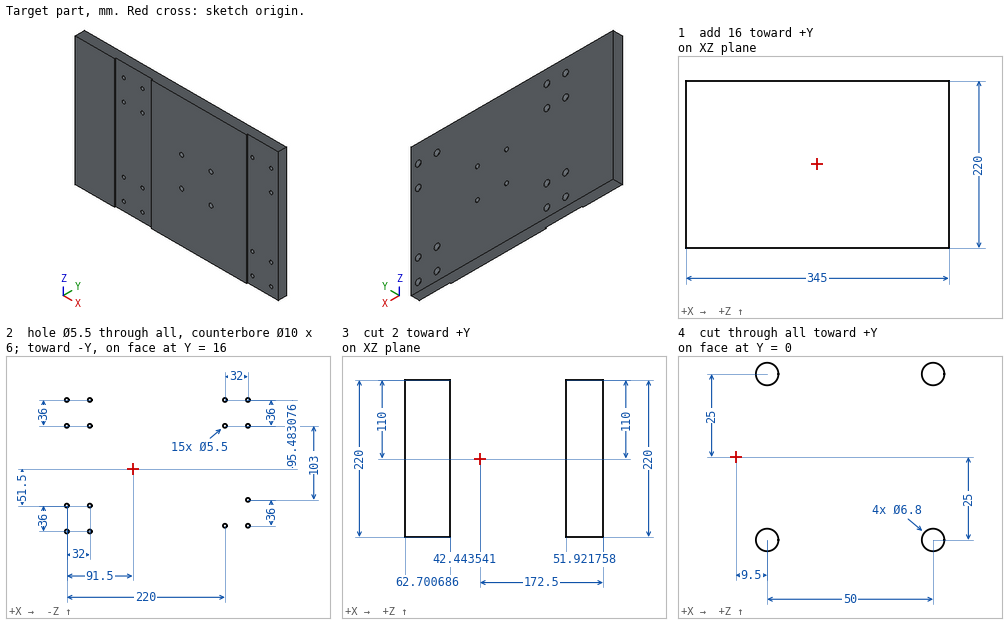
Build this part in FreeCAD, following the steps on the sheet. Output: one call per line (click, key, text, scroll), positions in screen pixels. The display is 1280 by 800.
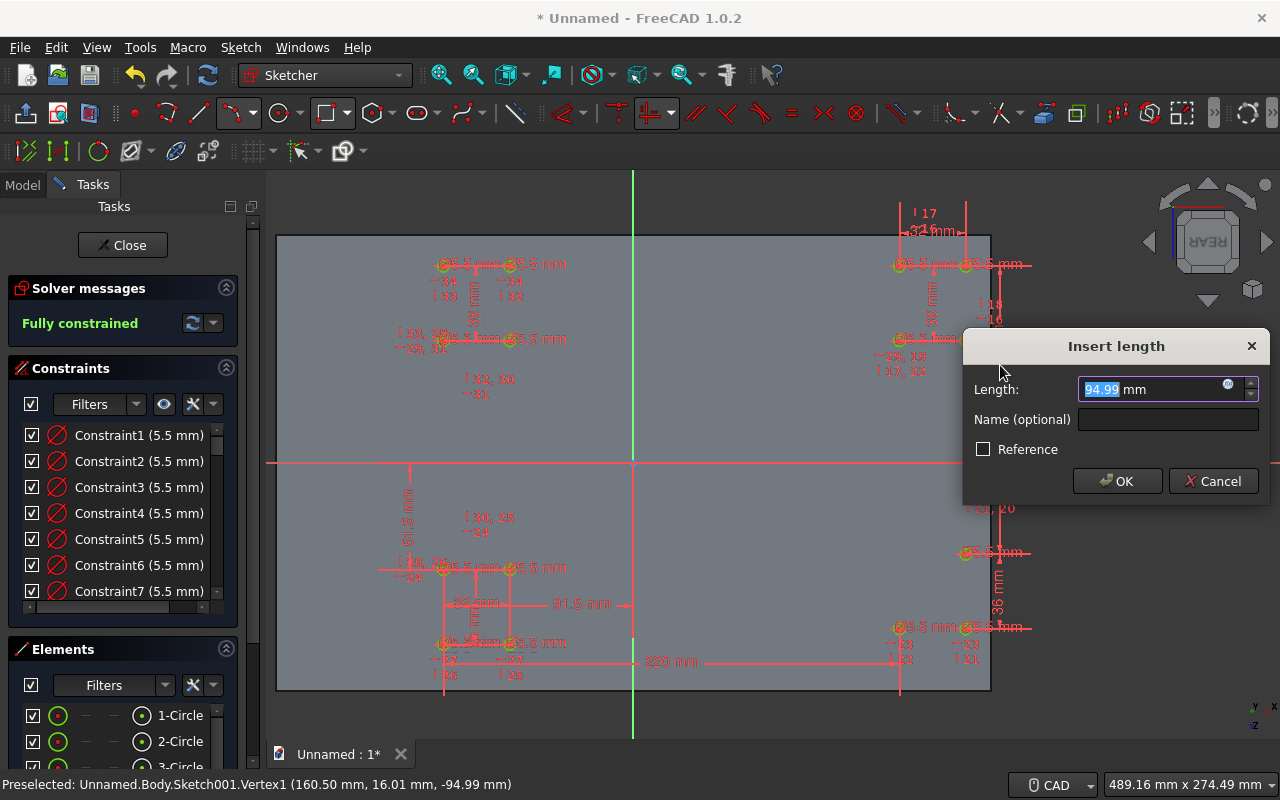
text(95.483076)
key(Return)
key(Escape)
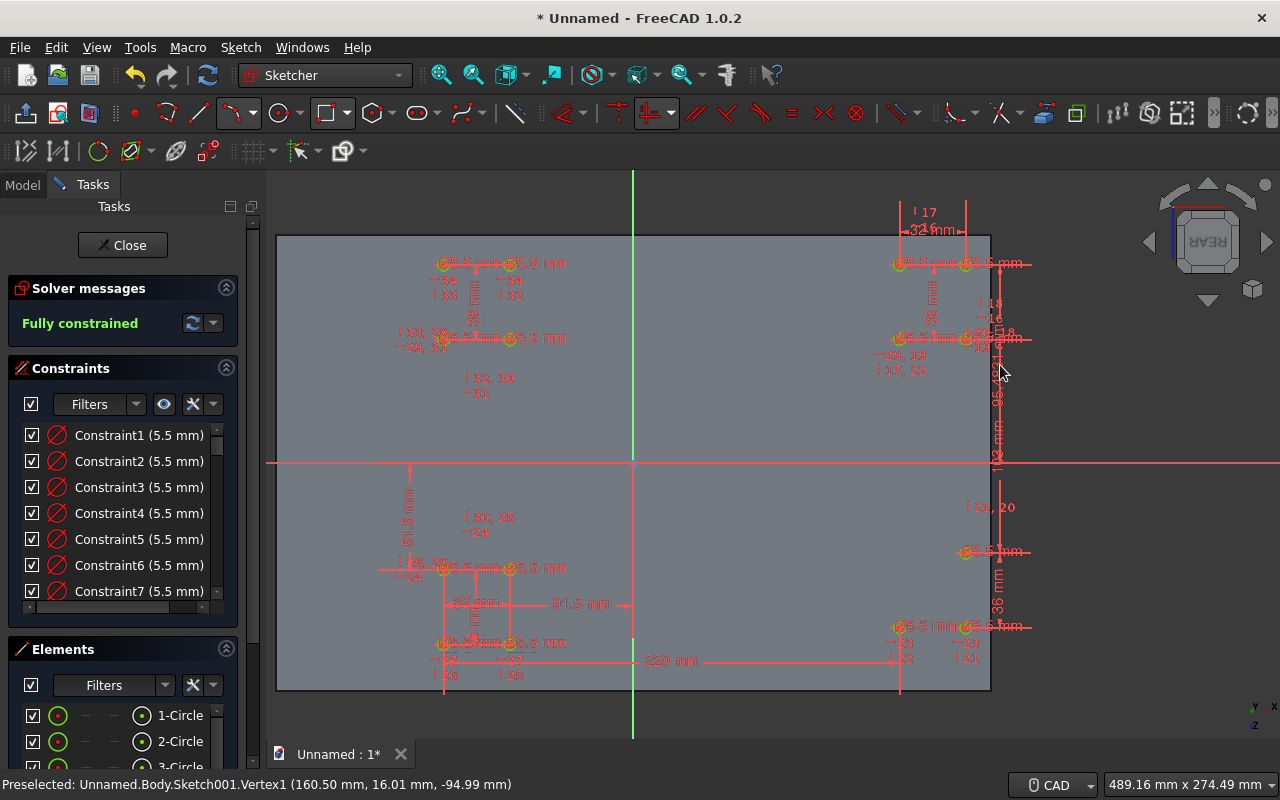
click(123, 245)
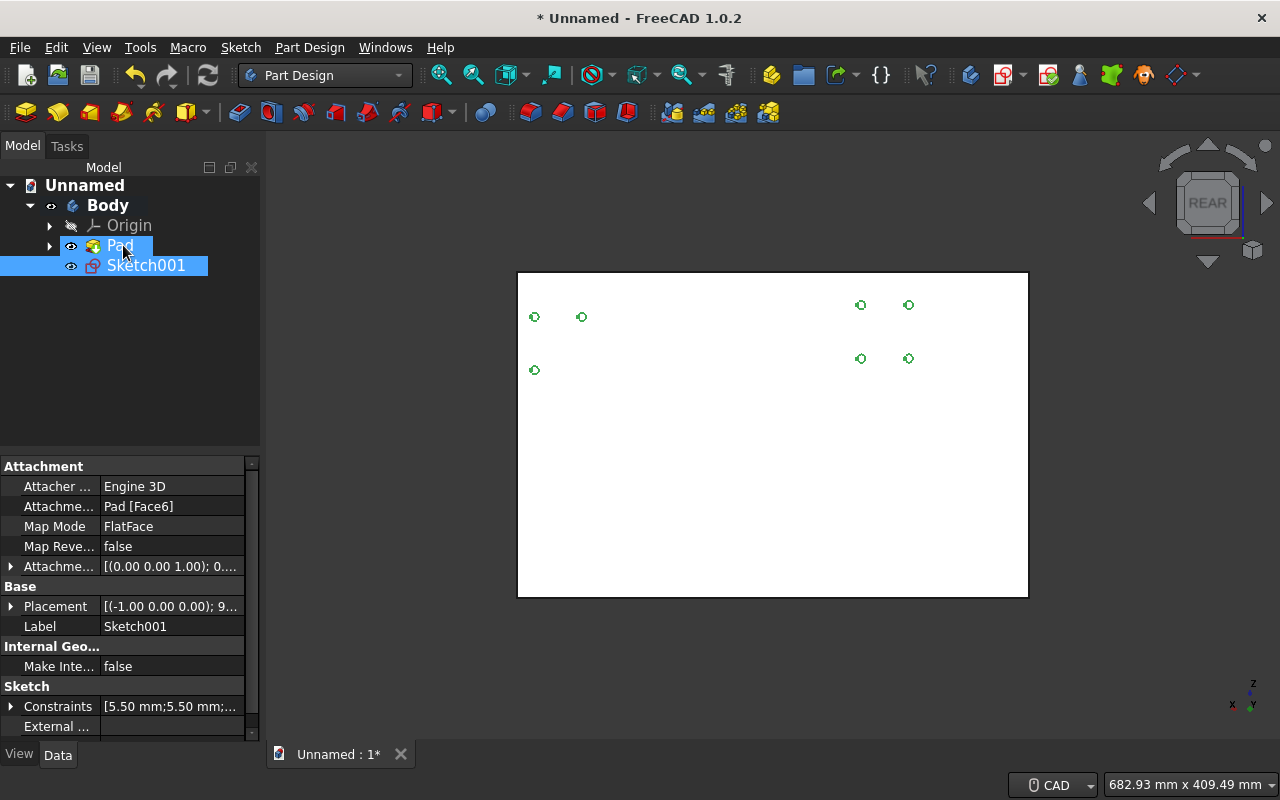
click(272, 112)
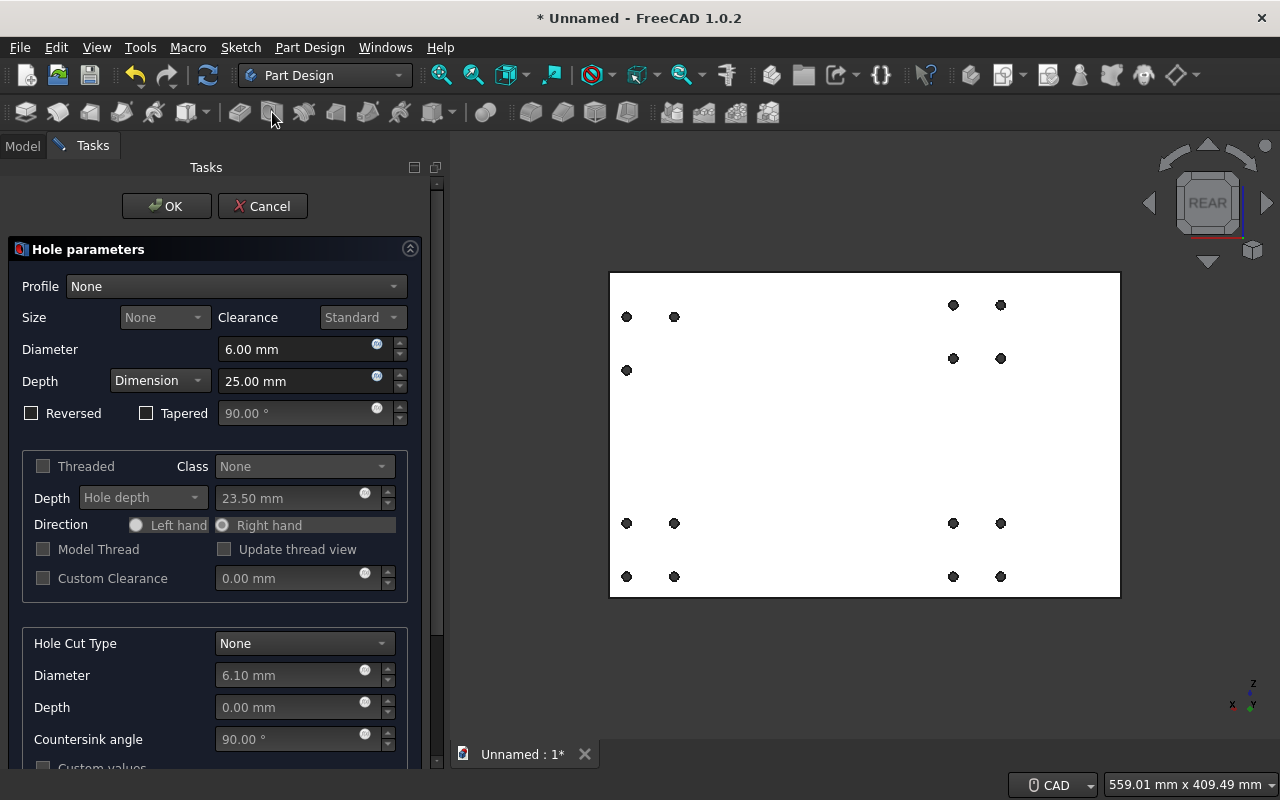
triple_click(305, 349)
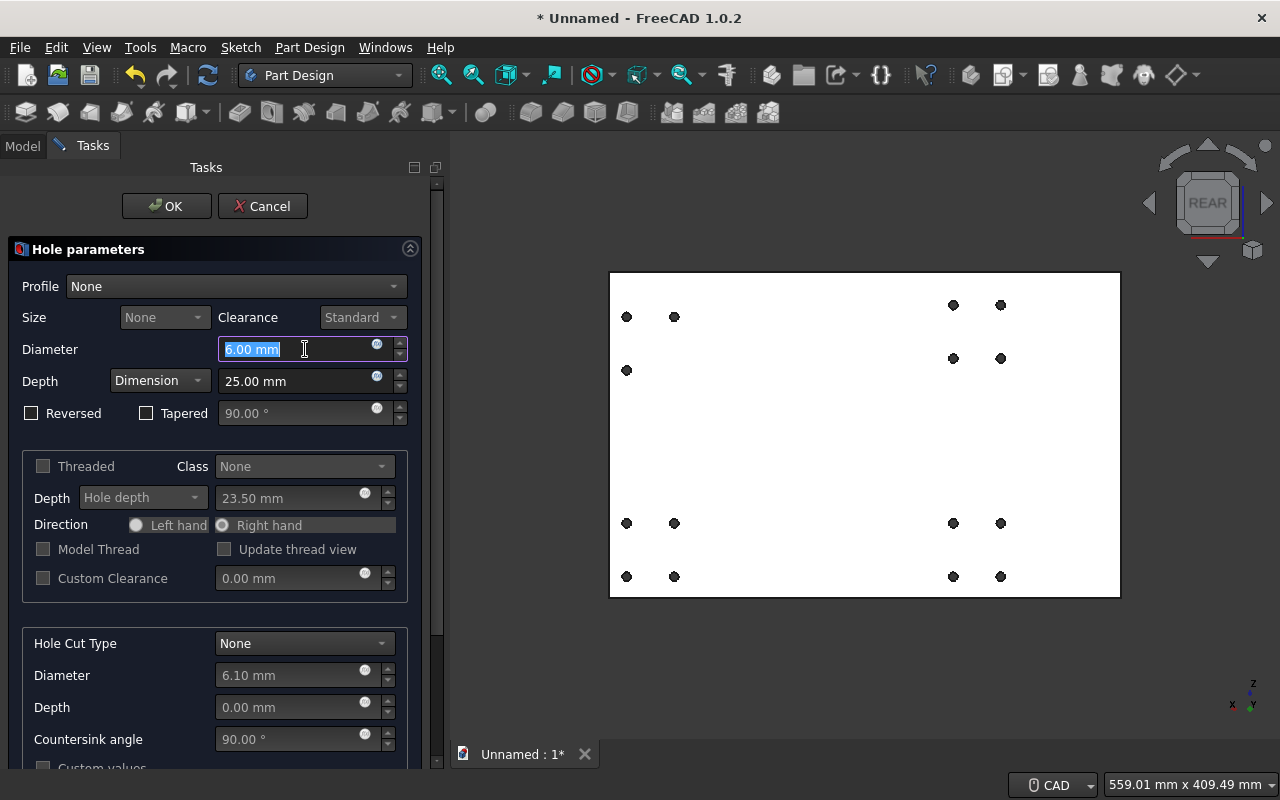
text(5.5)
key(Tab)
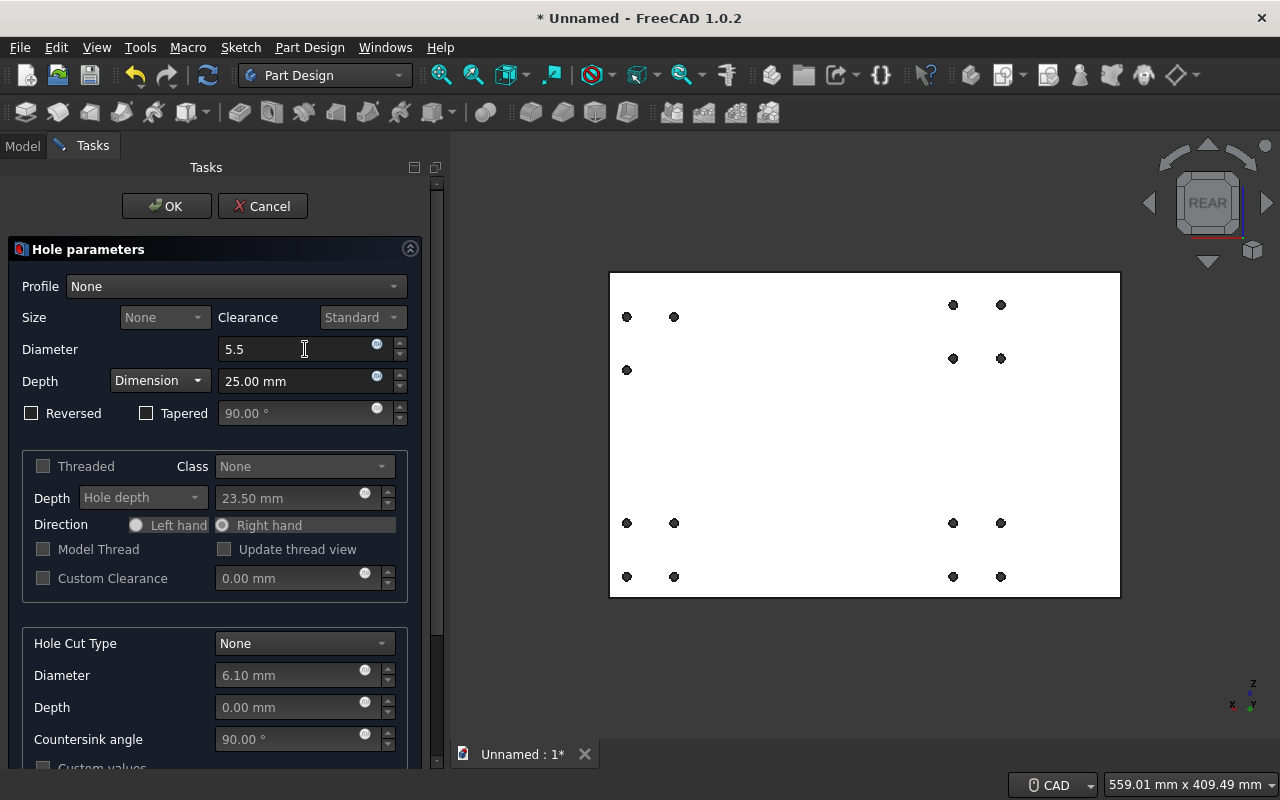
click(161, 380)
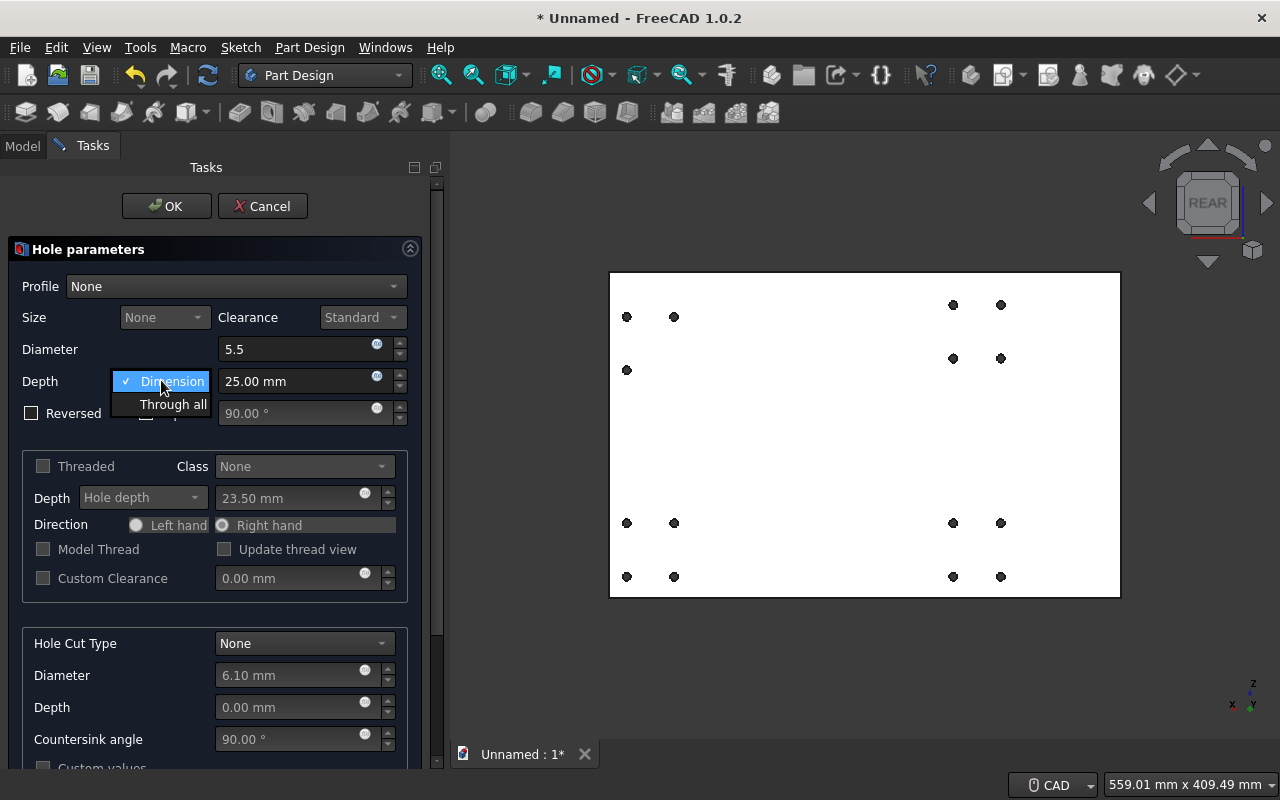
click(160, 404)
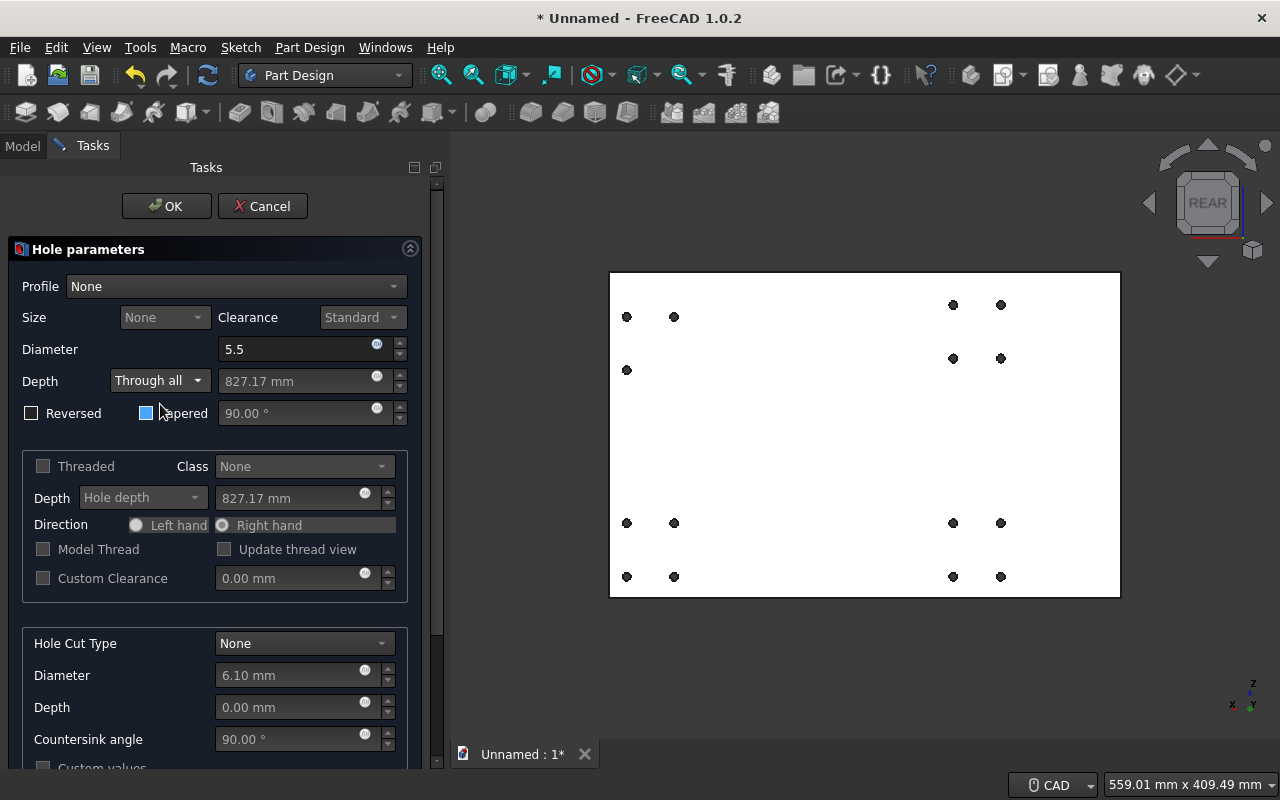
click(306, 644)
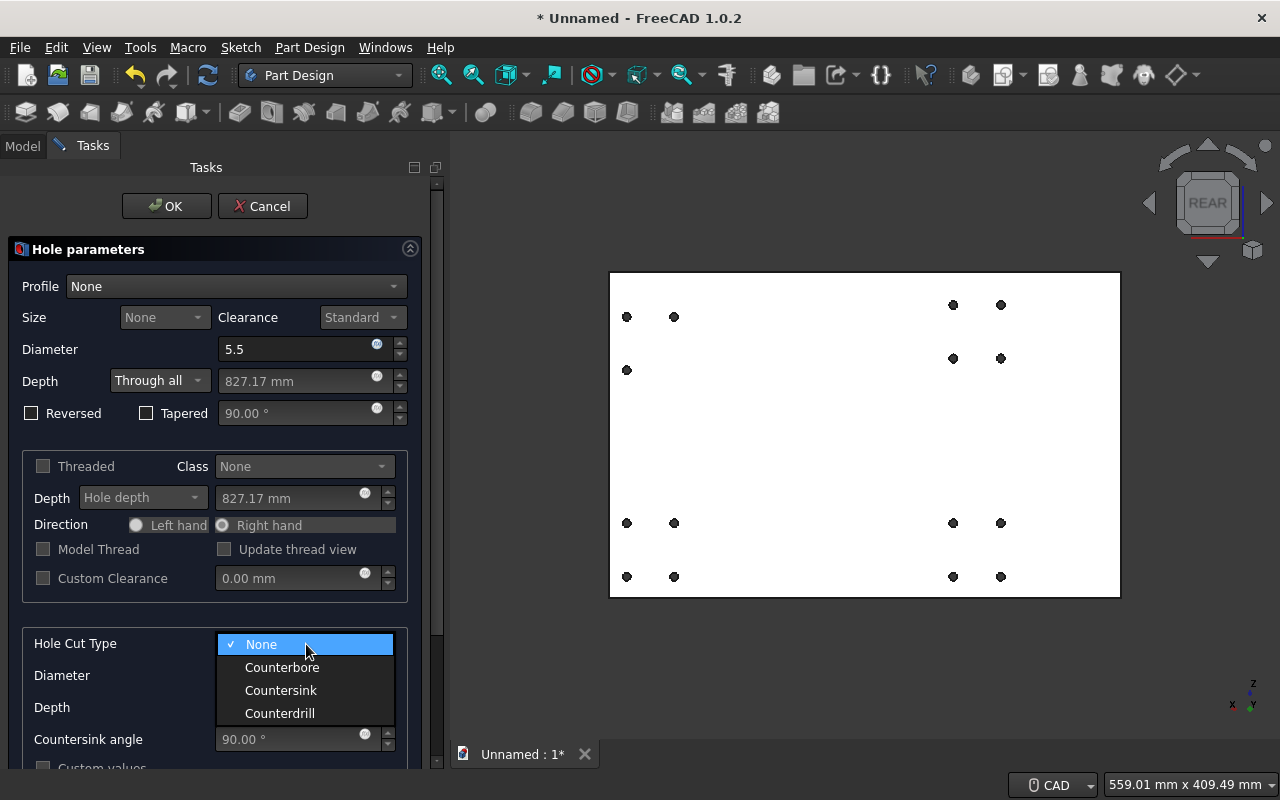
click(304, 668)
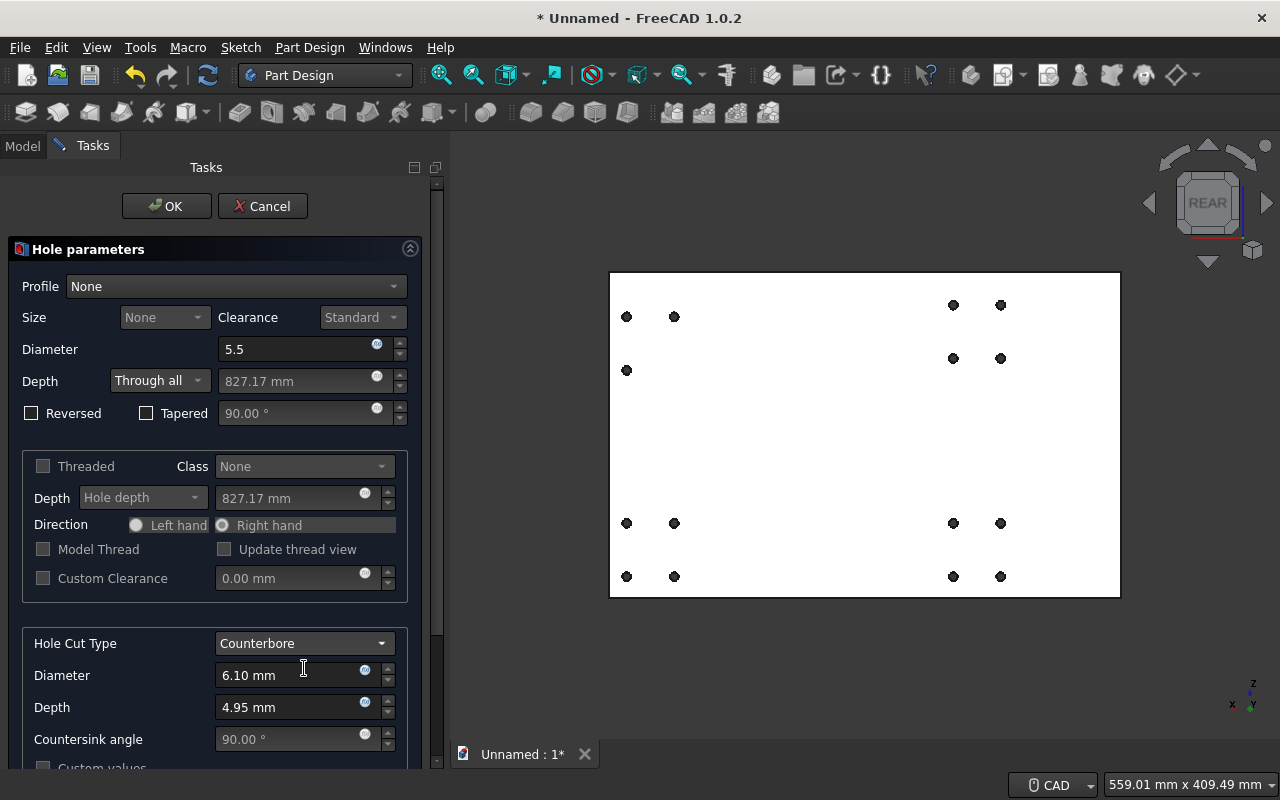
triple_click(298, 675)